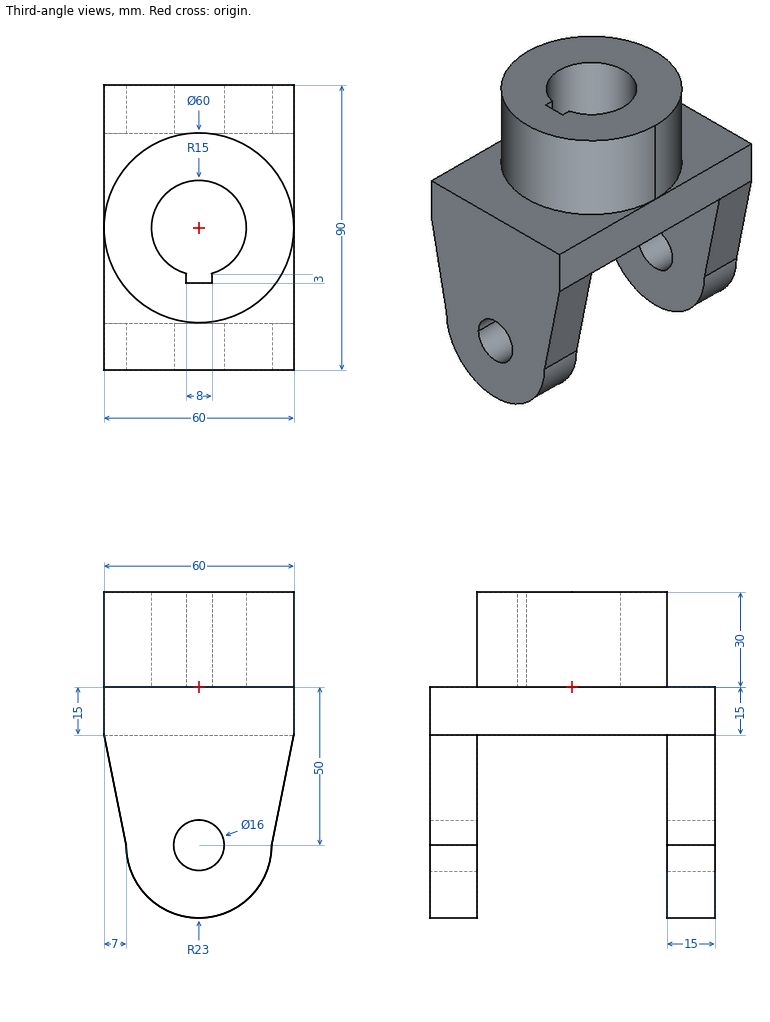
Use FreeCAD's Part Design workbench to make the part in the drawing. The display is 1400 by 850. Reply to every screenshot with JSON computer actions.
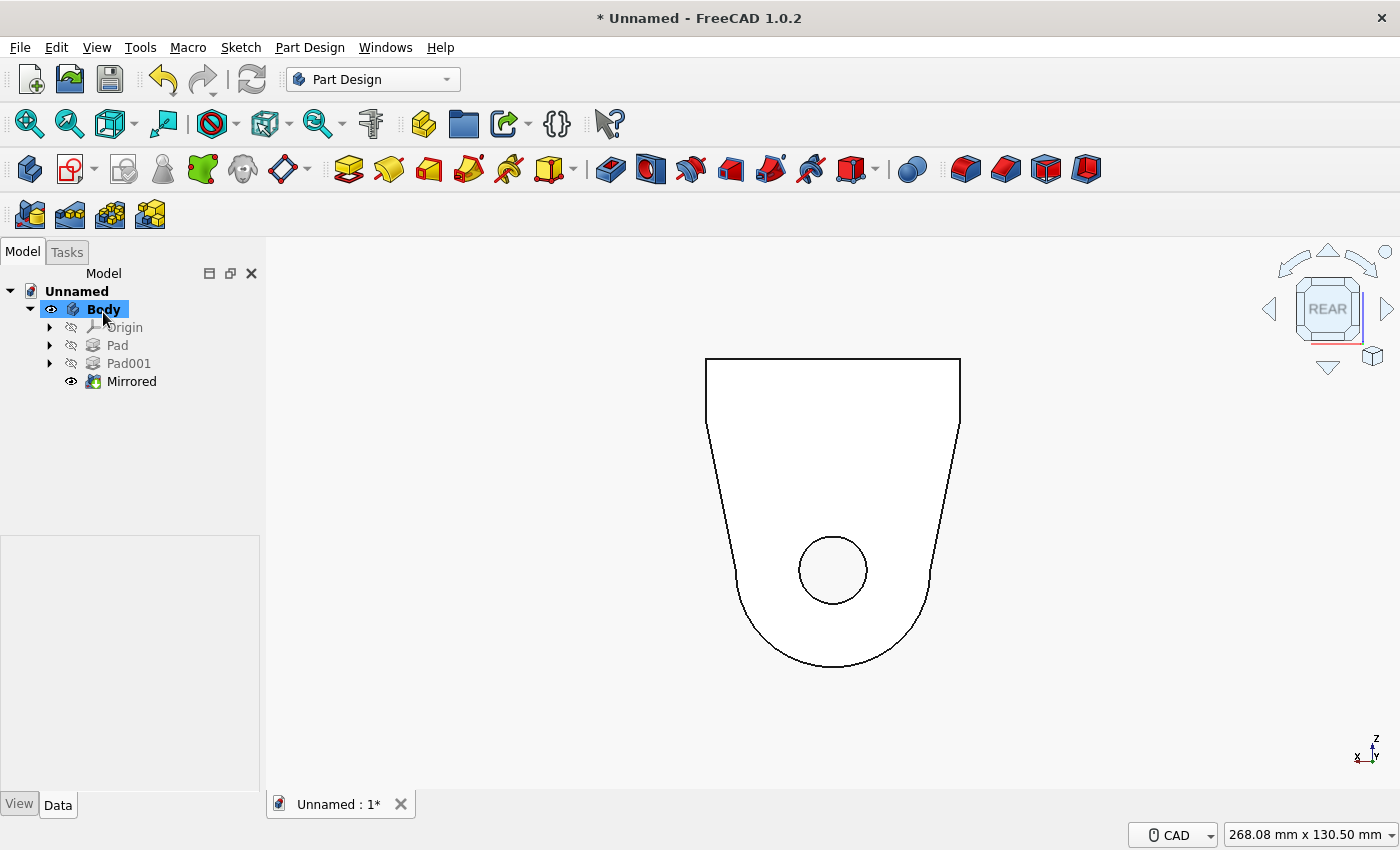
{"action": "key", "text": "0"}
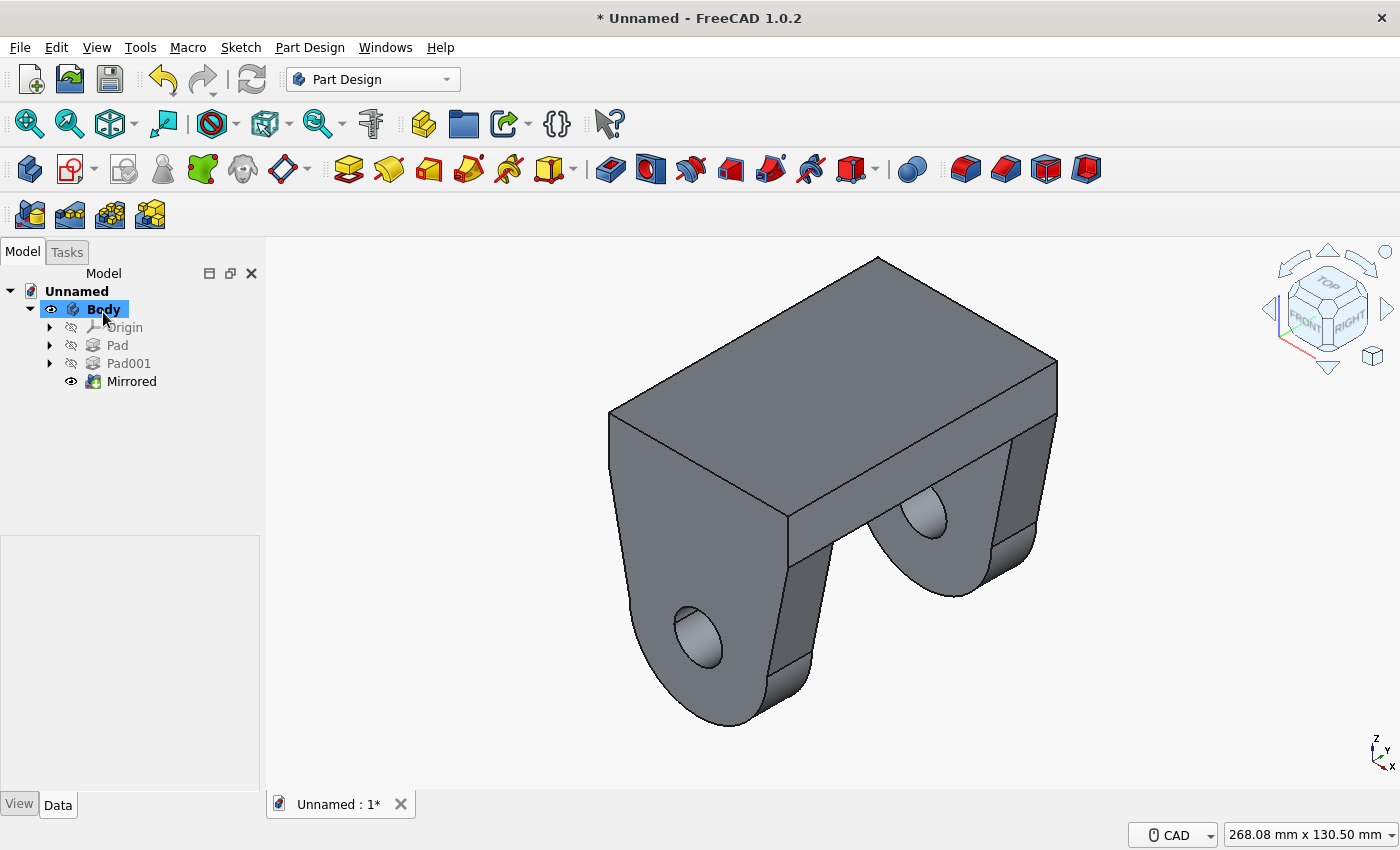
{"action": "left_click", "coordinate": [871, 364]}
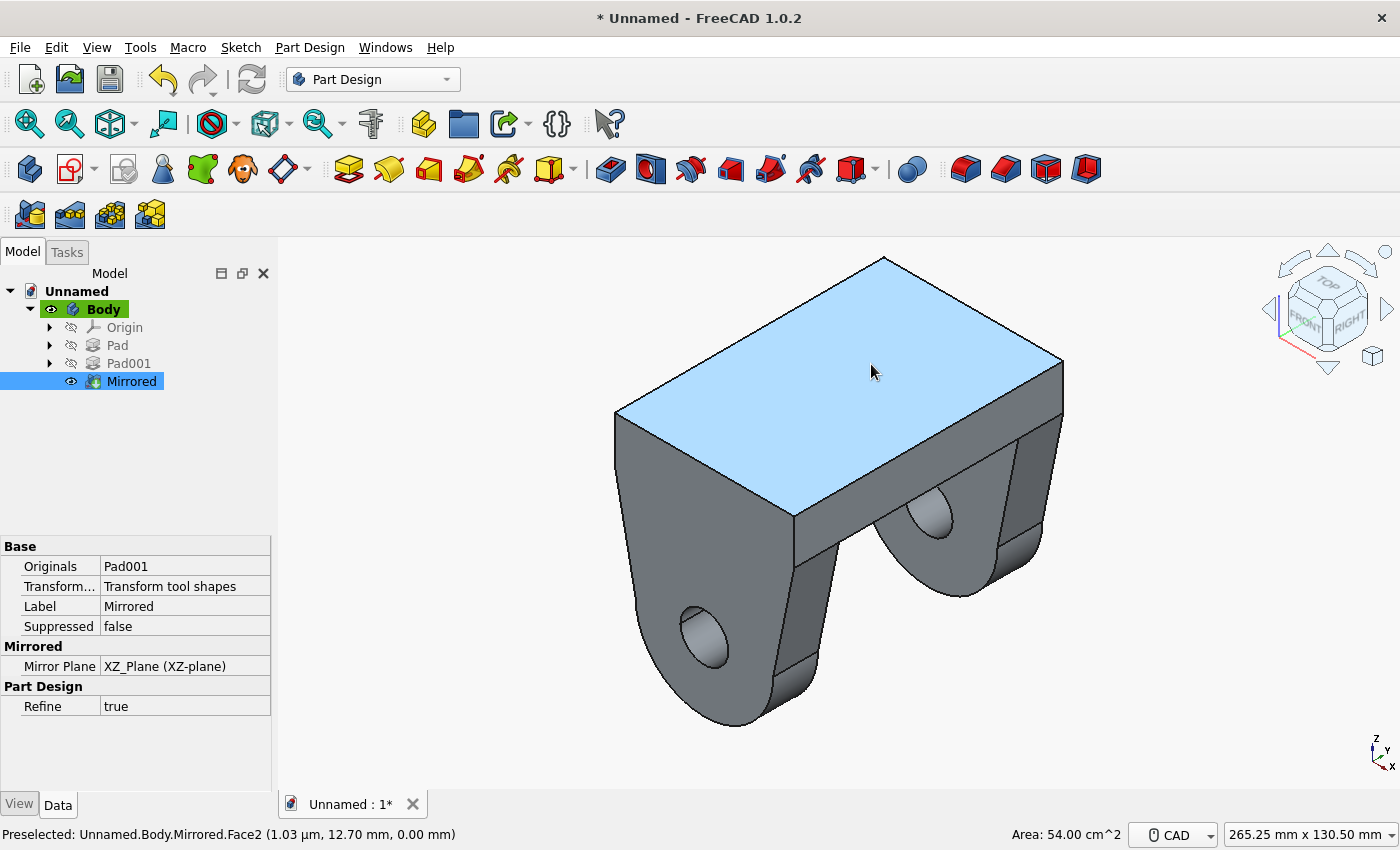
{"action": "left_click", "coordinate": [70, 170]}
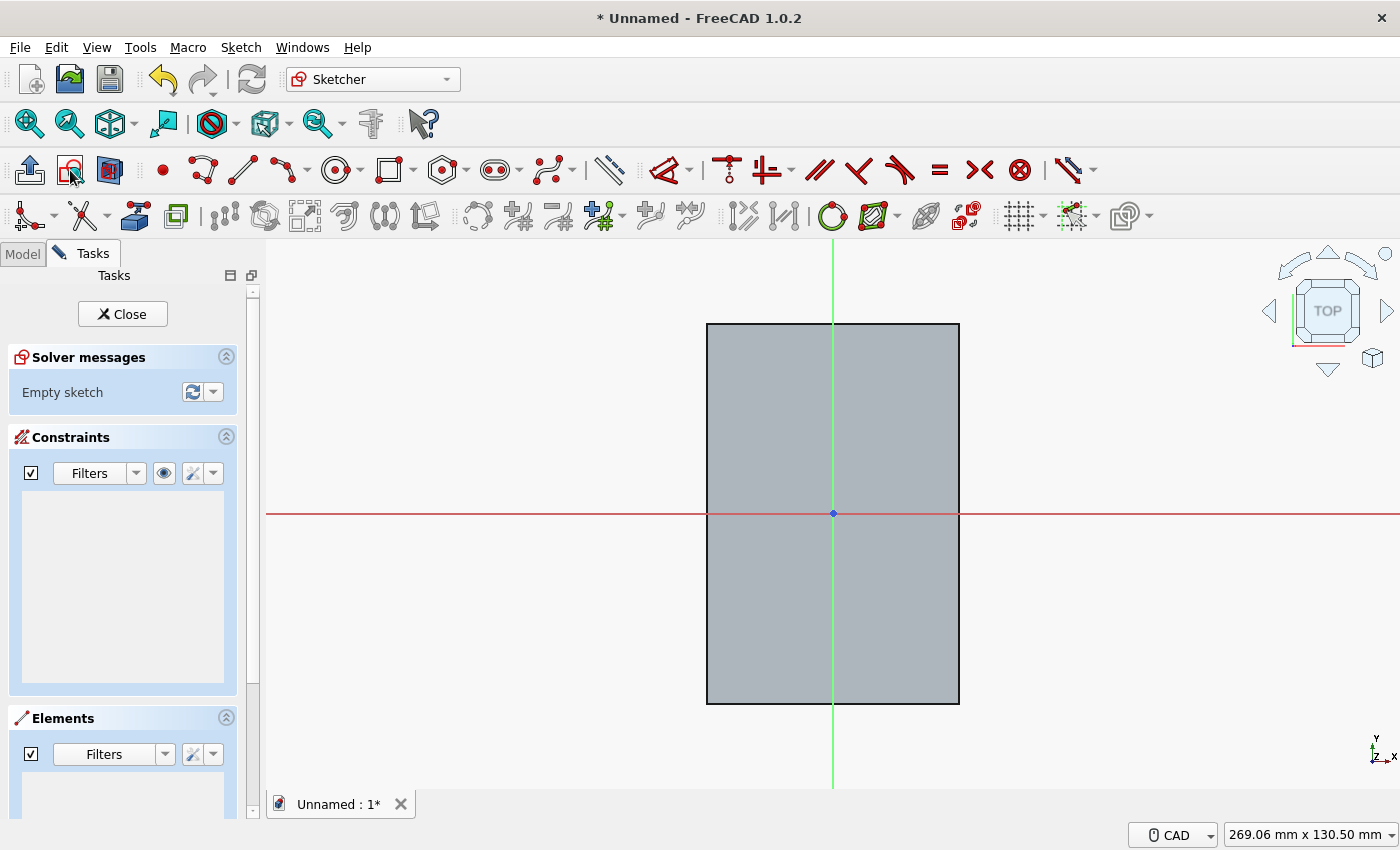
{"action": "scroll", "coordinate": [972, 514], "scroll_direction": "up", "scroll_amount": 2}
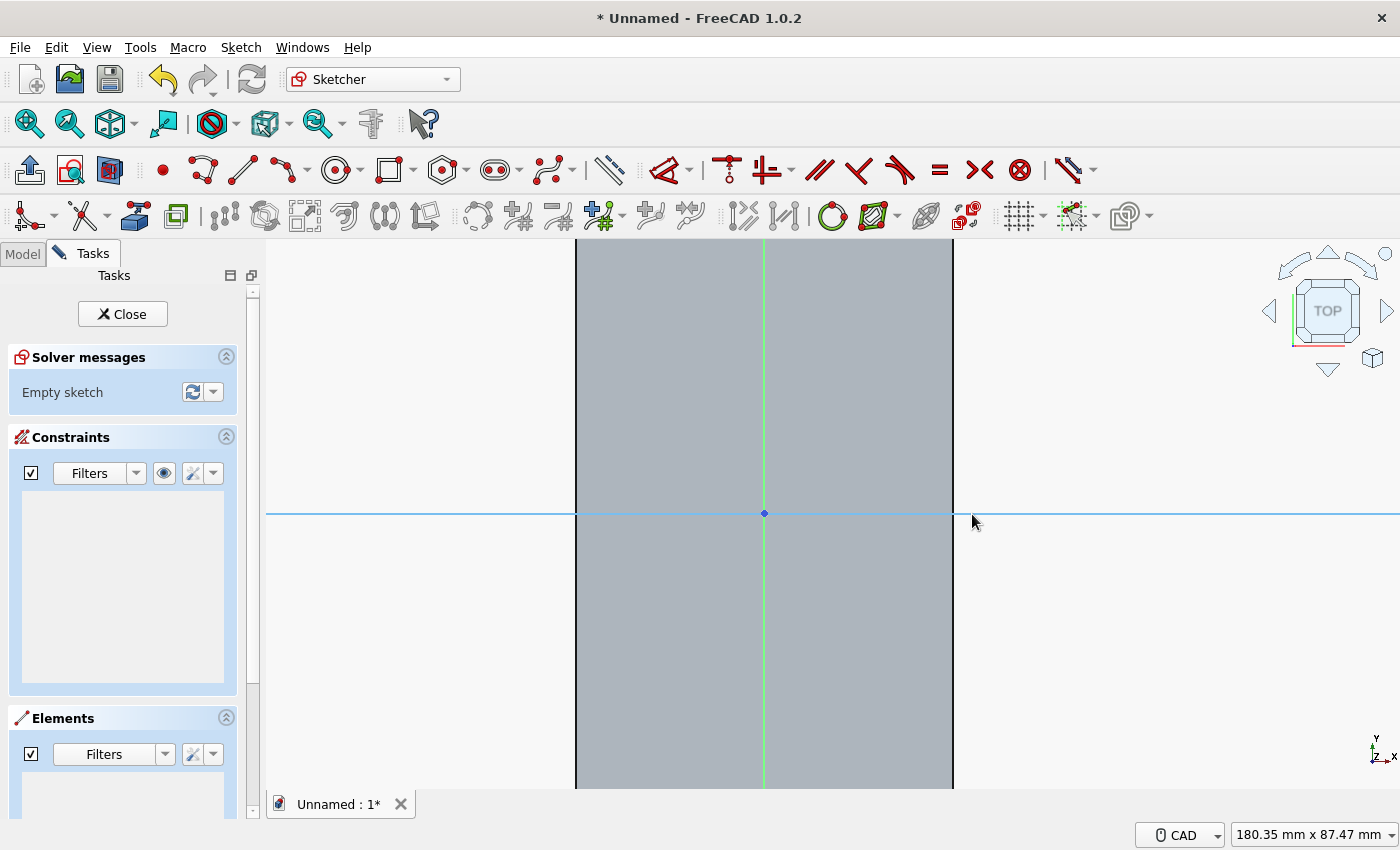
{"action": "left_click", "coordinate": [204, 170]}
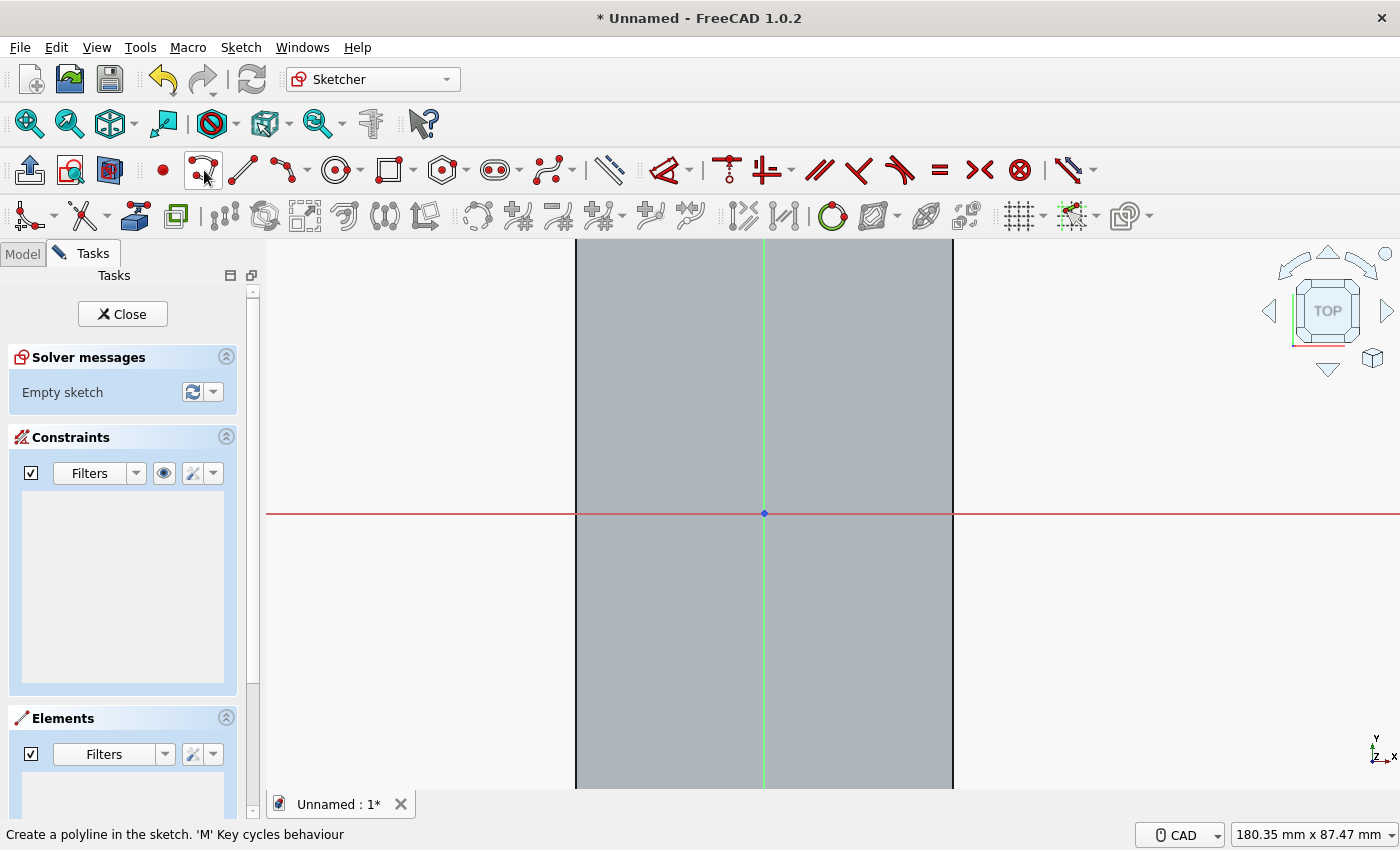
{"action": "left_click", "coordinate": [789, 605]}
{"action": "left_click", "coordinate": [789, 624]}
{"action": "left_click", "coordinate": [739, 624]}
{"action": "left_click", "coordinate": [739, 605]}
{"action": "right_click", "coordinate": [739, 605]}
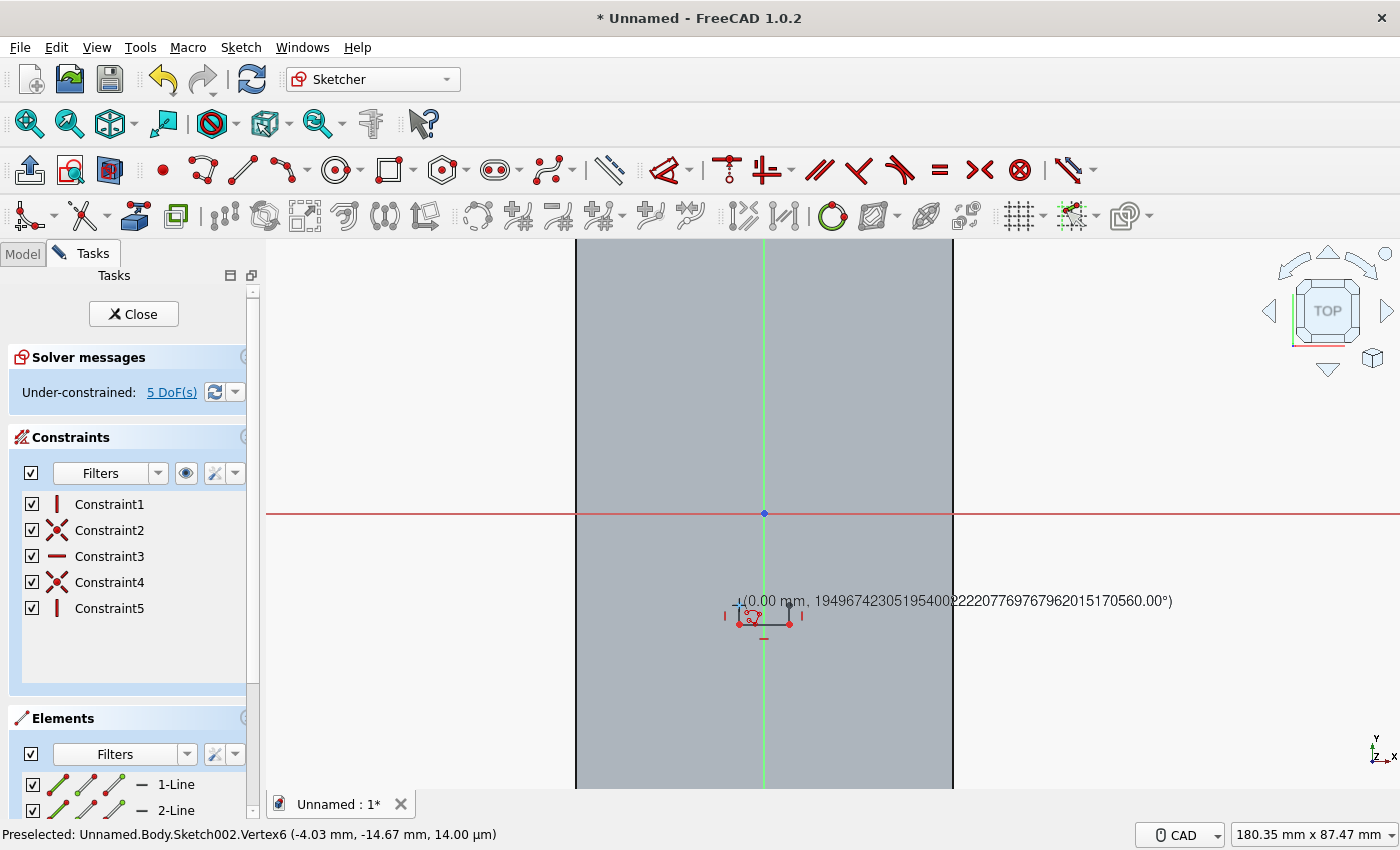
{"action": "left_click", "coordinate": [284, 170]}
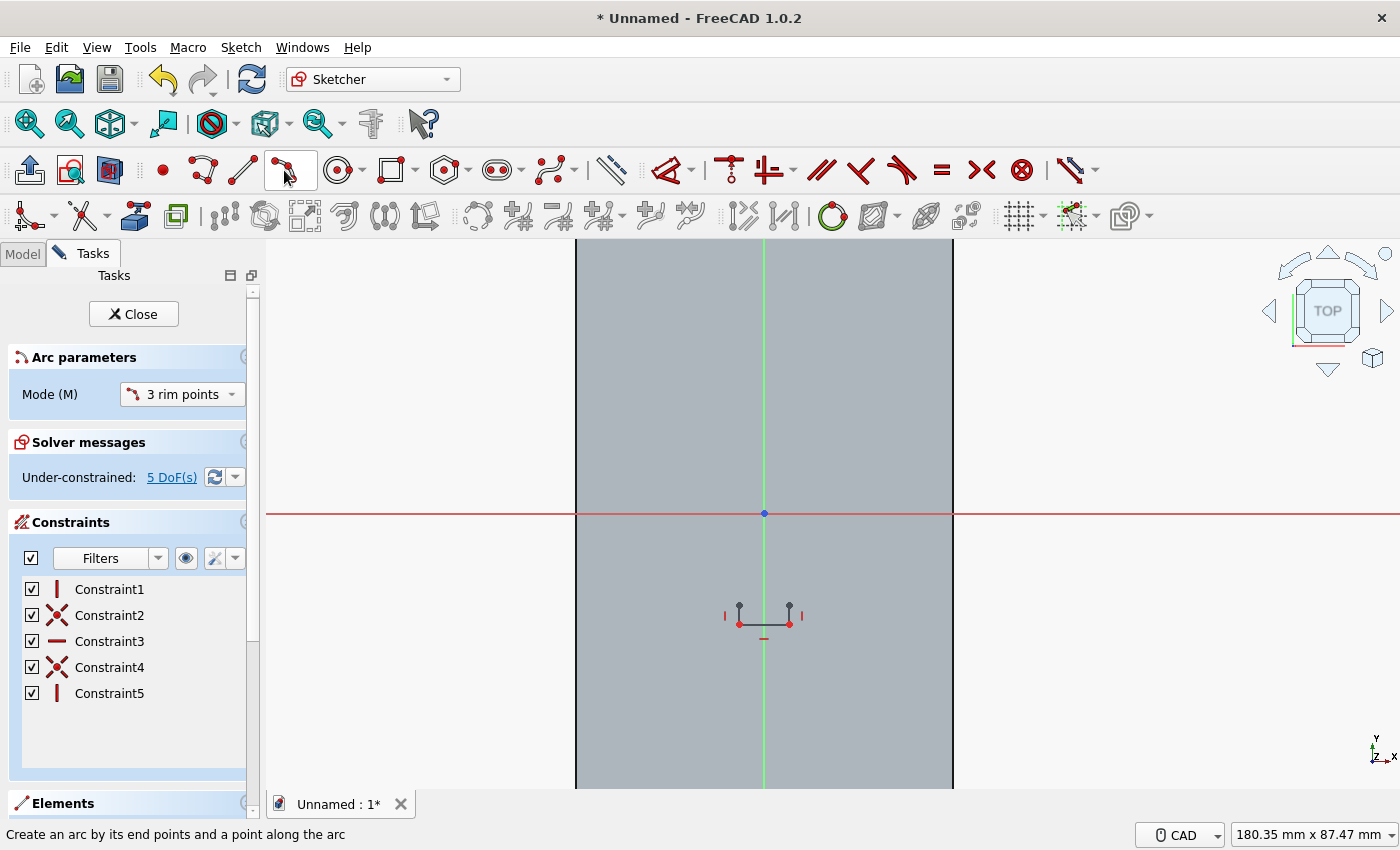
{"action": "scroll", "coordinate": [739, 605], "scroll_direction": "up", "scroll_amount": 3}